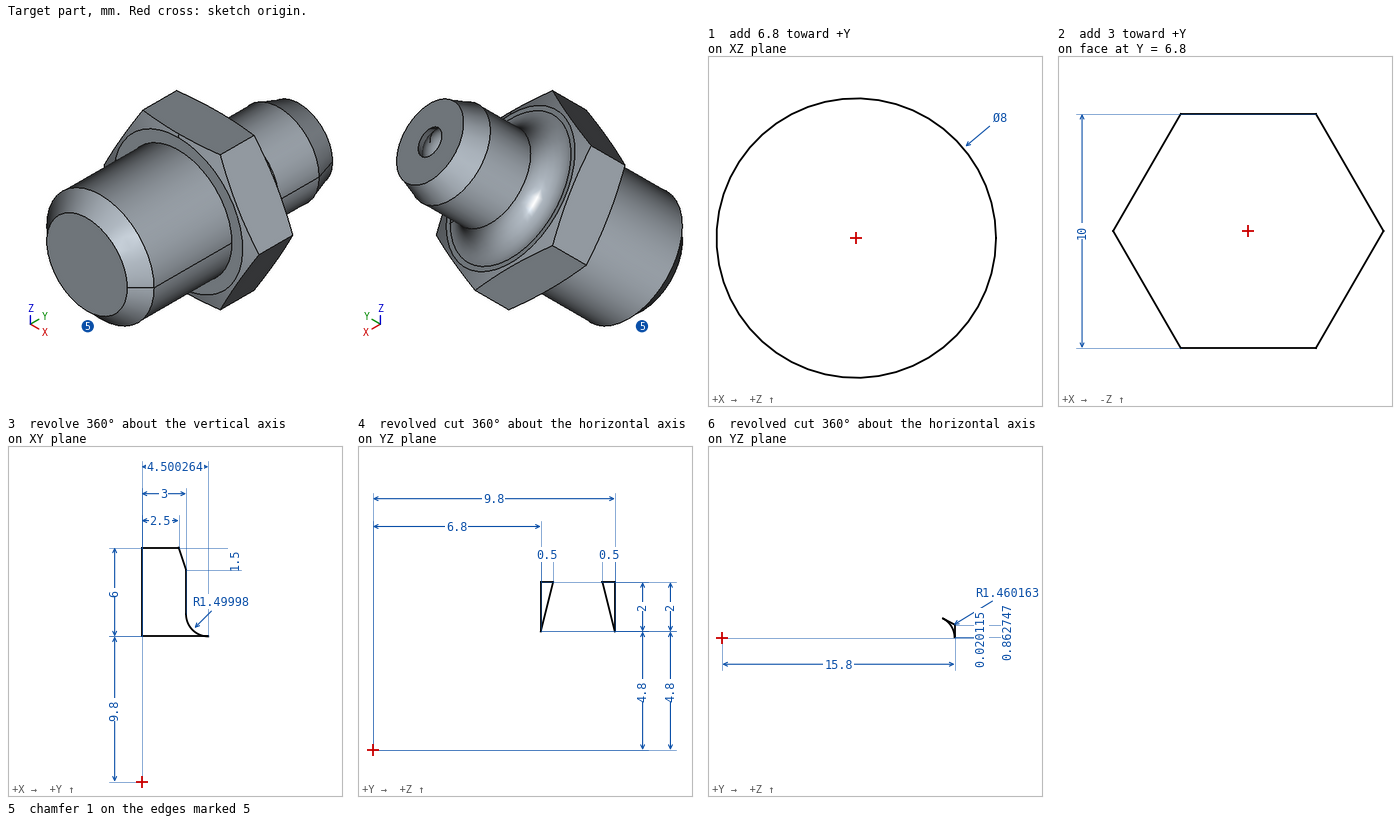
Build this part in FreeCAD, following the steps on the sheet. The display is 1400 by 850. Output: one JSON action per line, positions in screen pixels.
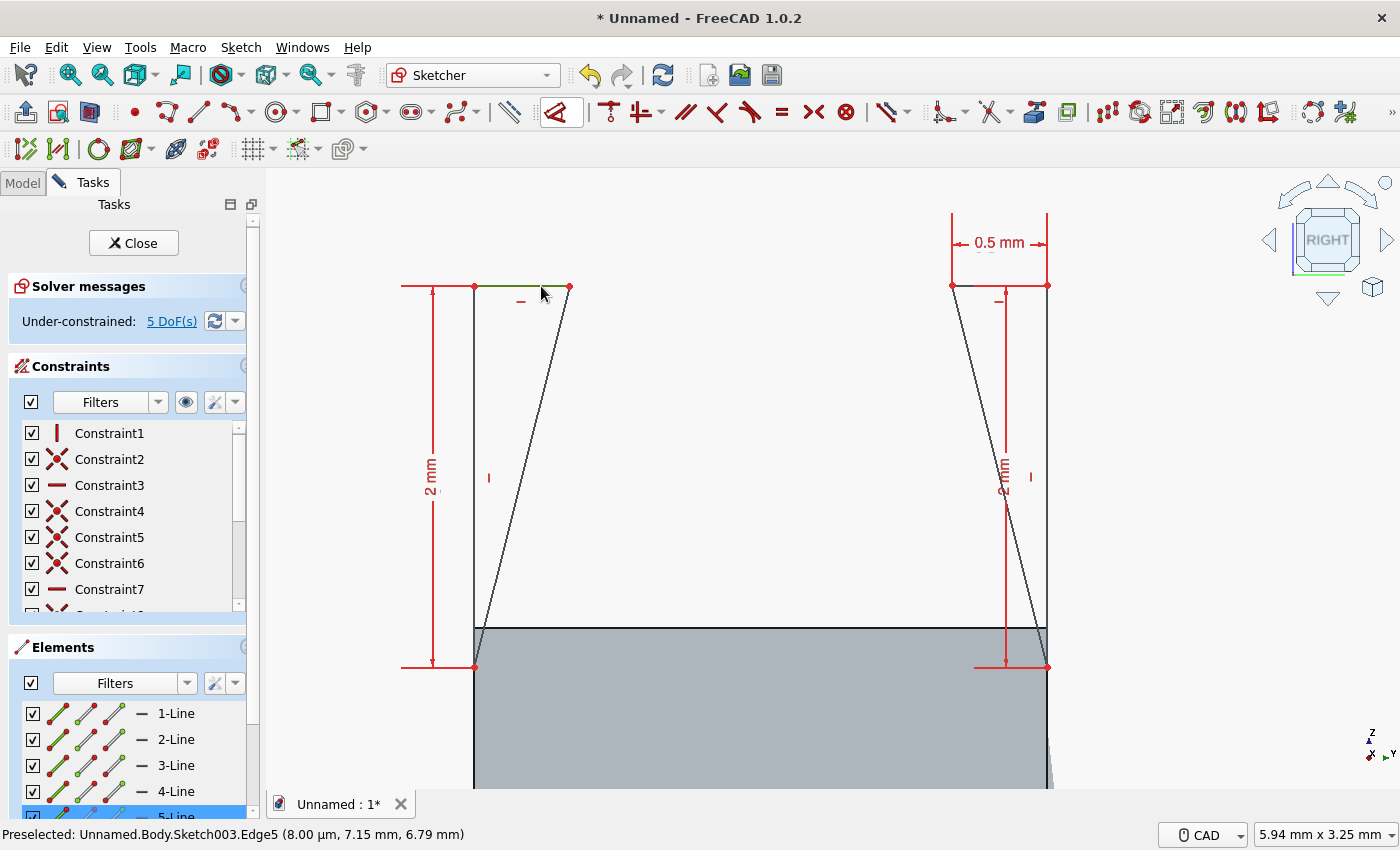
{"action": "key", "text": "l"}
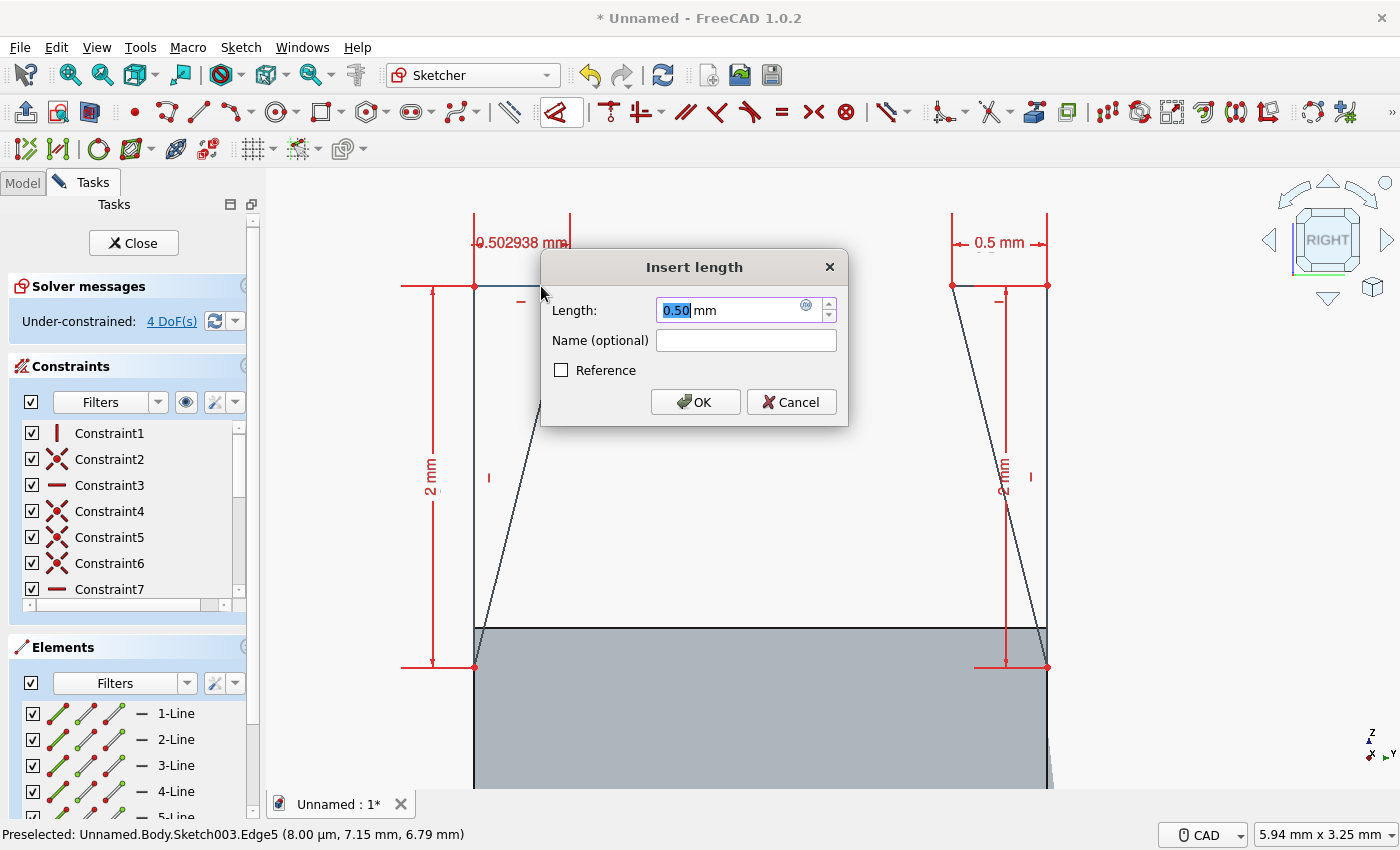
{"action": "type", "text": "0.5"}
{"action": "key", "text": "Return"}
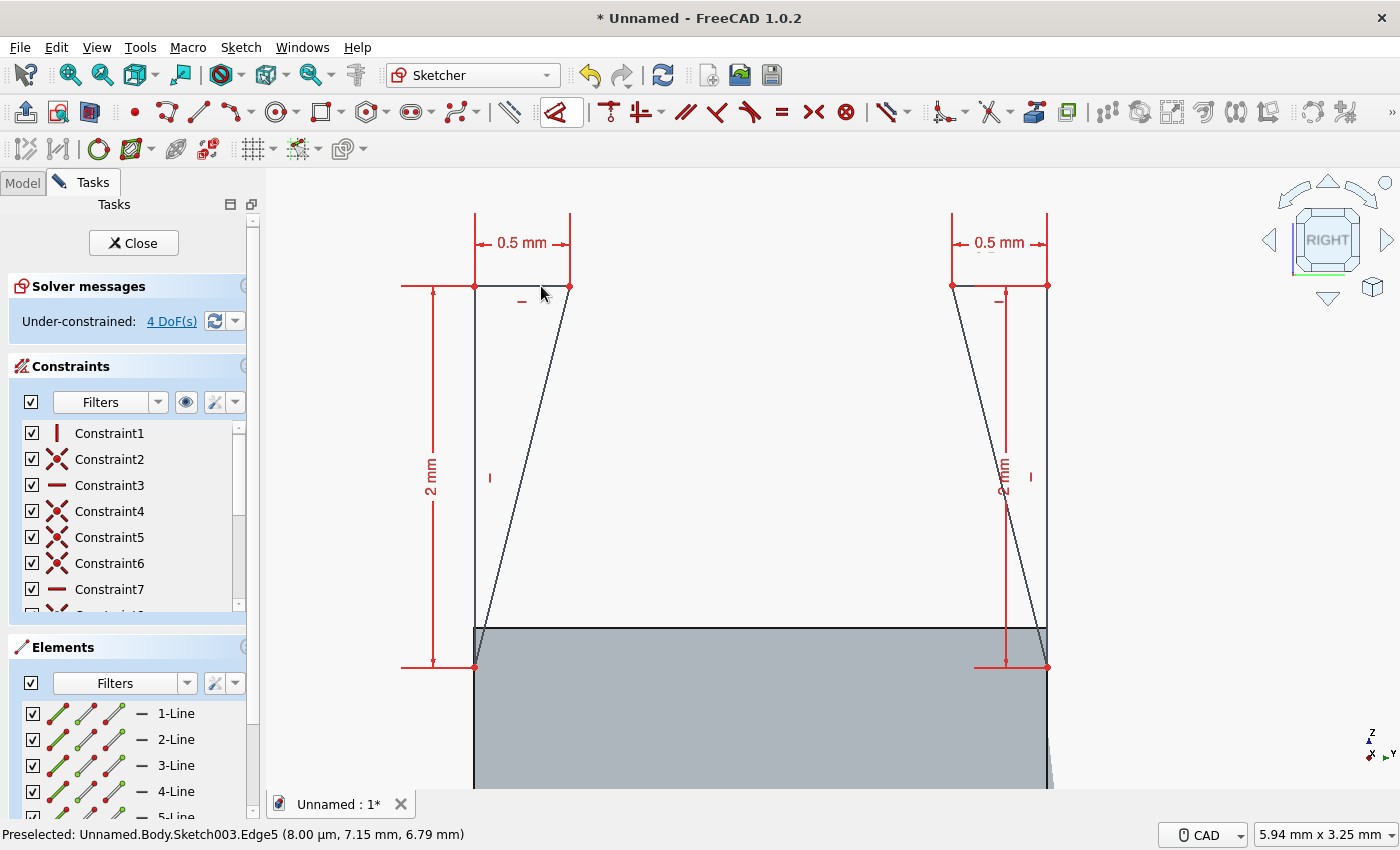
{"action": "left_click", "coordinate": [1047, 668]}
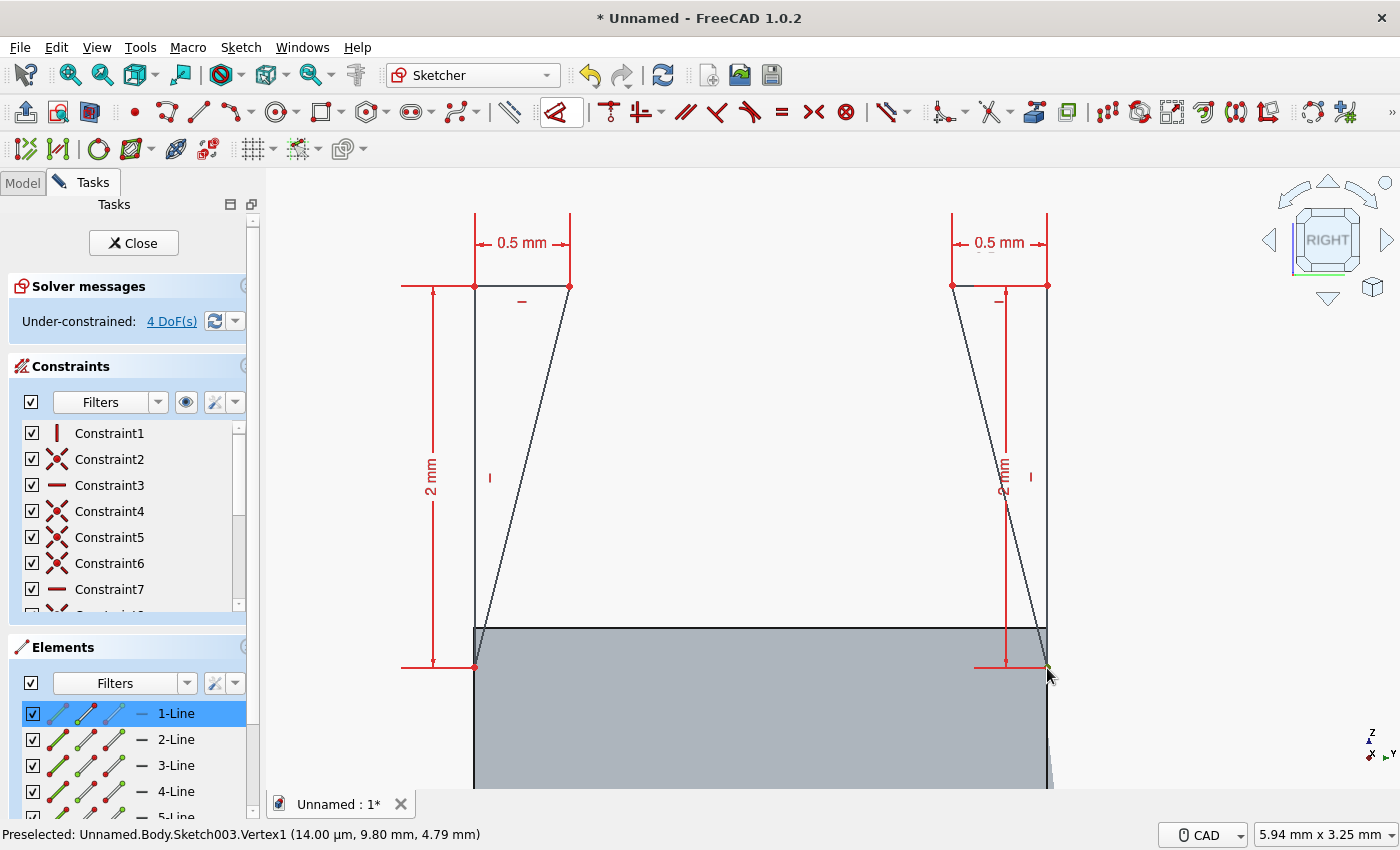
{"action": "key", "text": "l"}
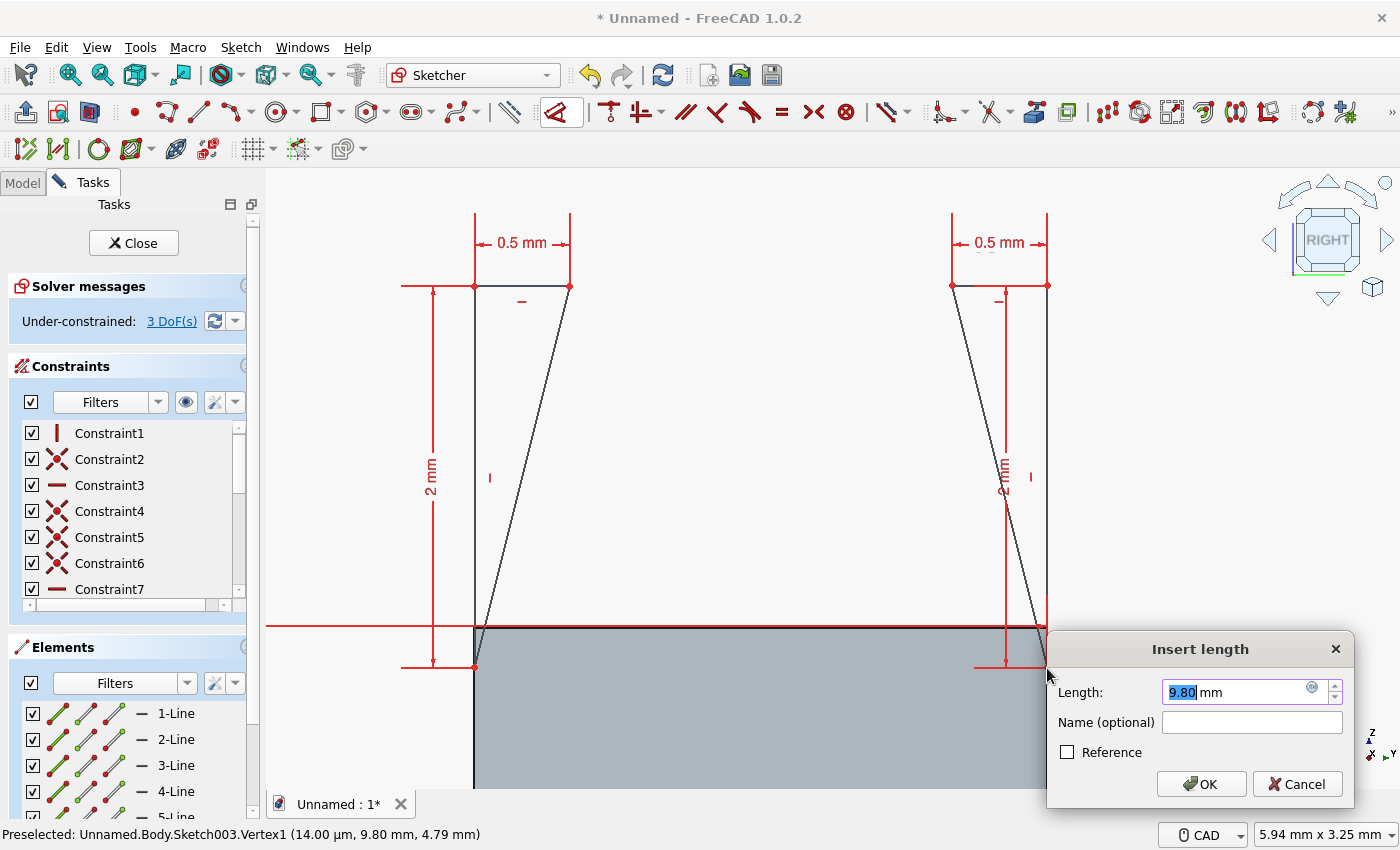
{"action": "type", "text": "9.8"}
{"action": "key", "text": "Return"}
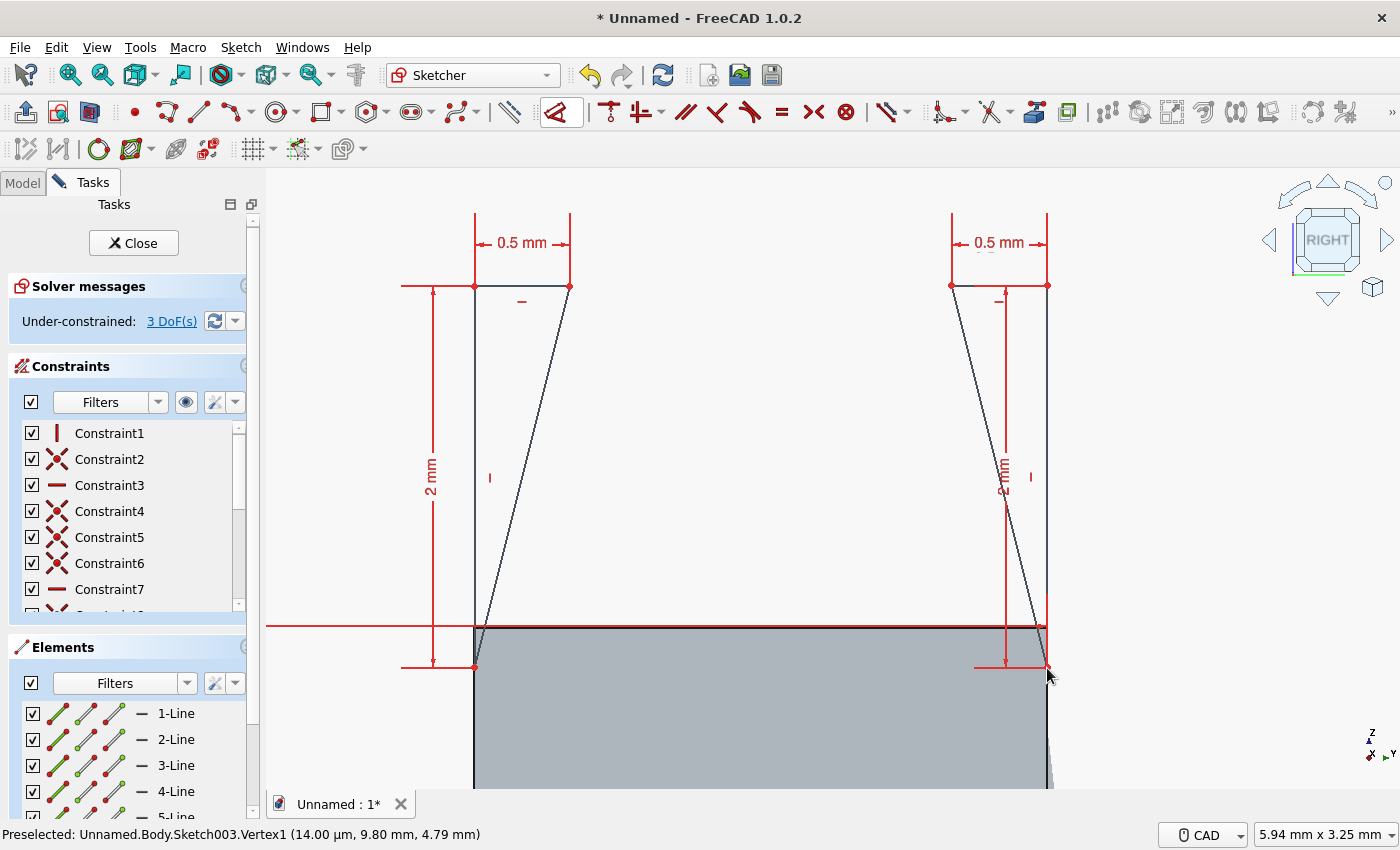
{"action": "left_click", "coordinate": [1047, 668]}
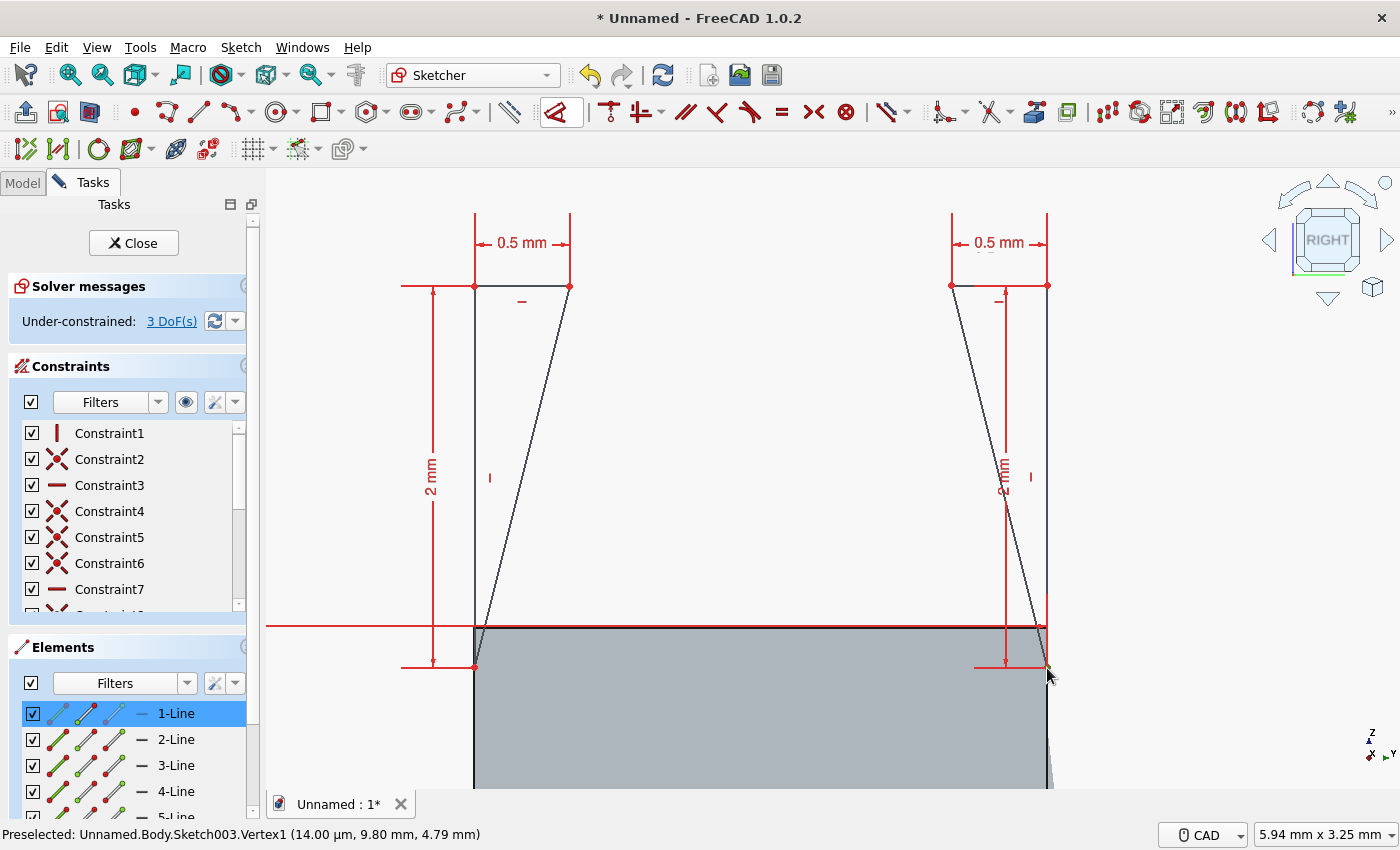
{"action": "key", "text": "i"}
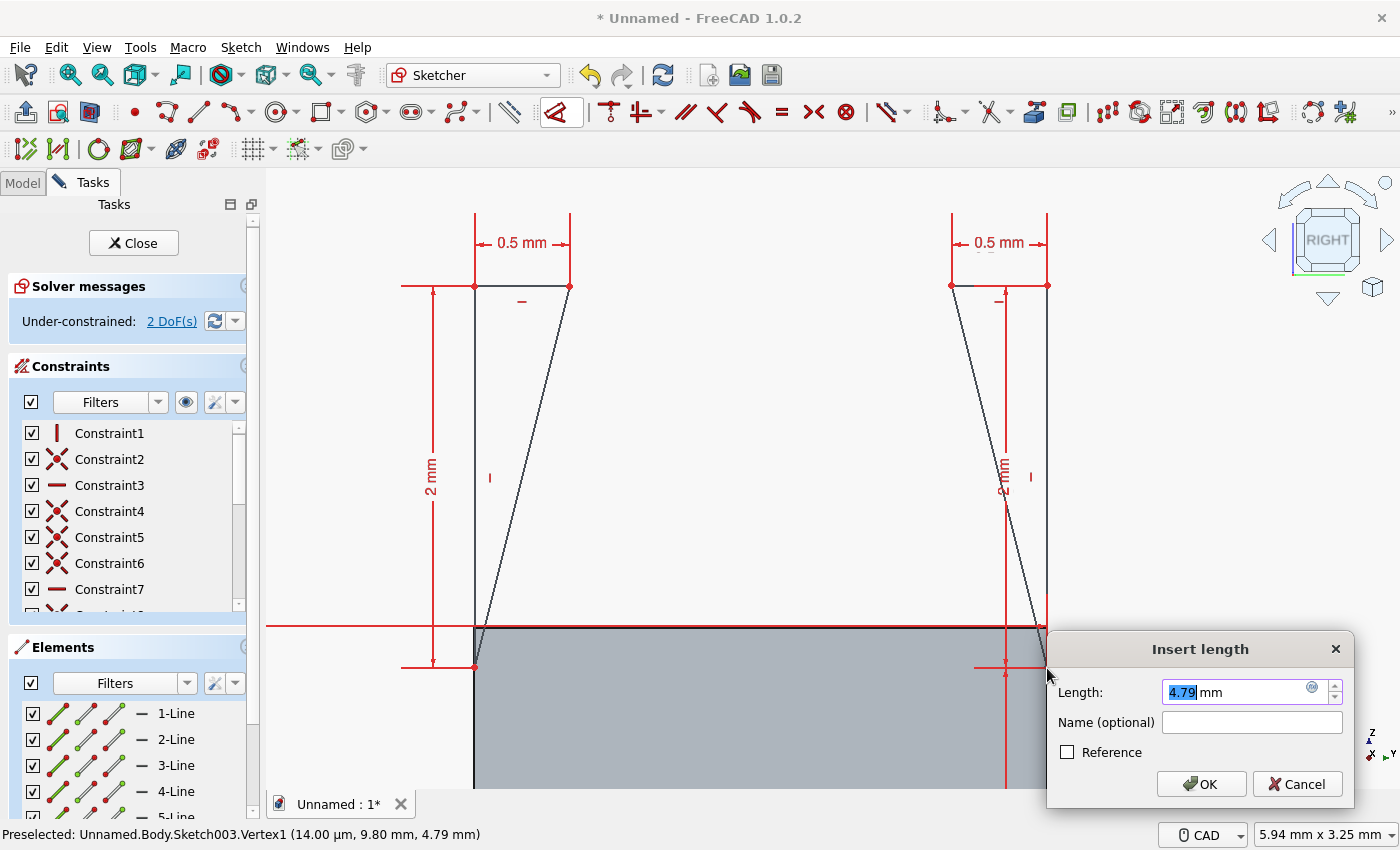
{"action": "type", "text": "4.8"}
{"action": "key", "text": "Return"}